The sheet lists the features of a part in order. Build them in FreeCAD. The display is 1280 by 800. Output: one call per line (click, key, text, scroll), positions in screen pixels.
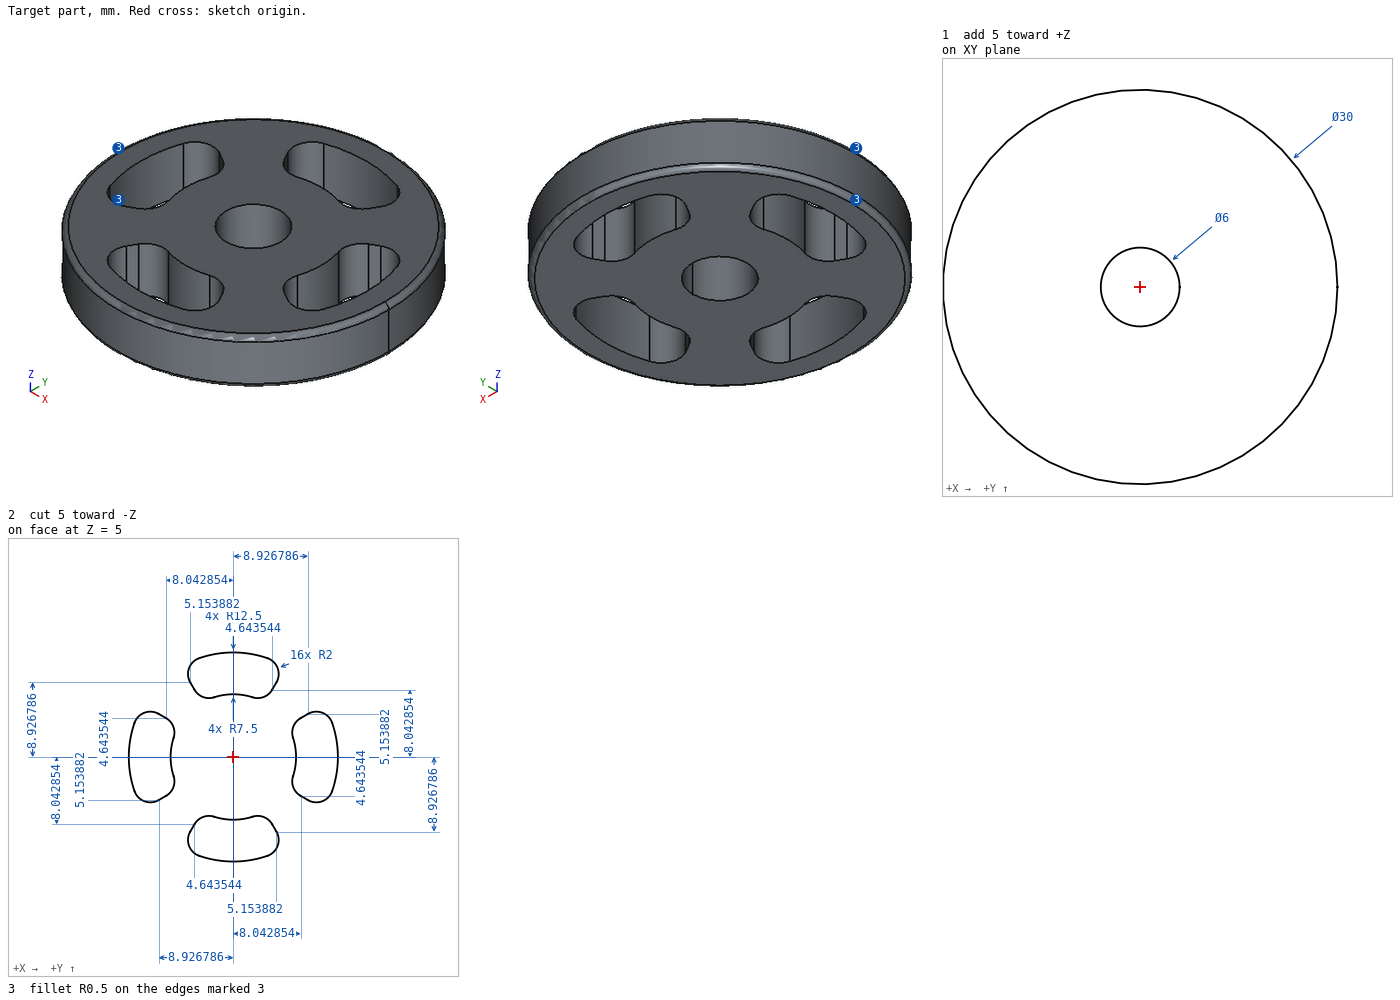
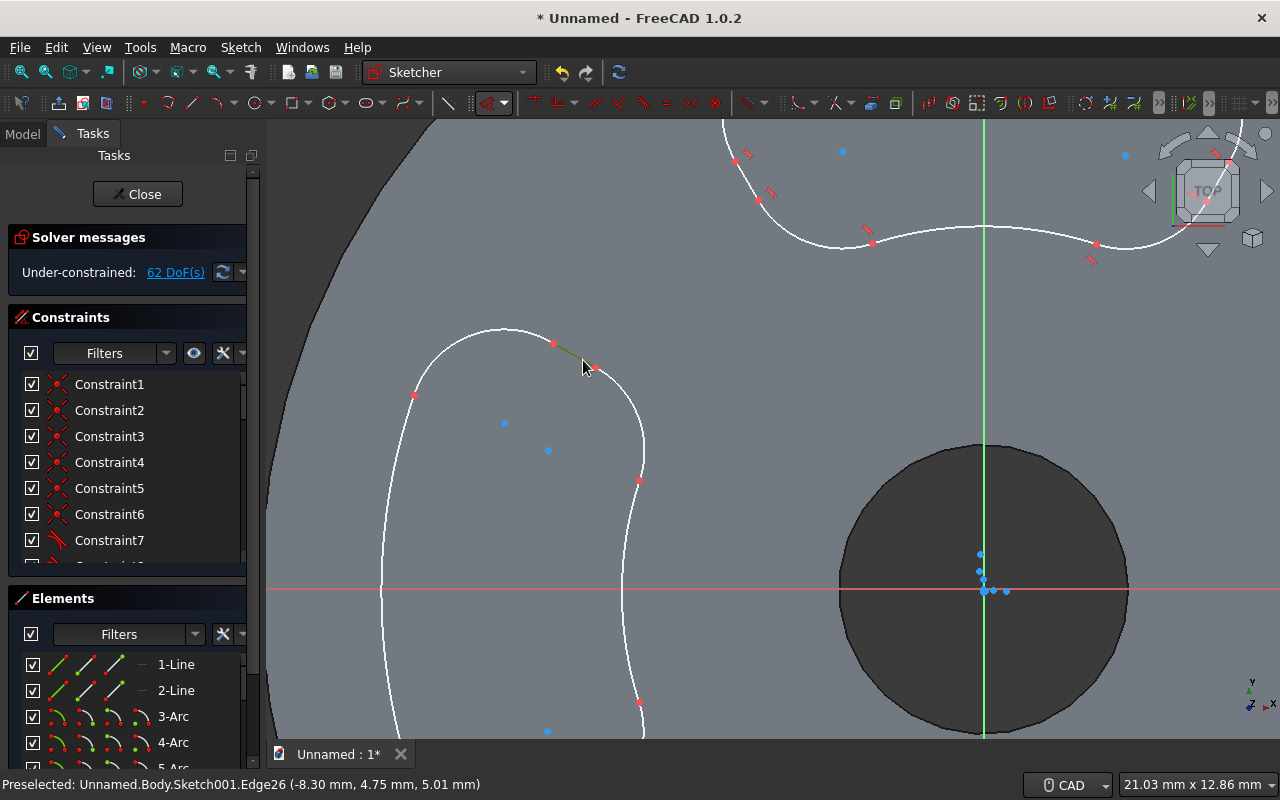
click(644, 441)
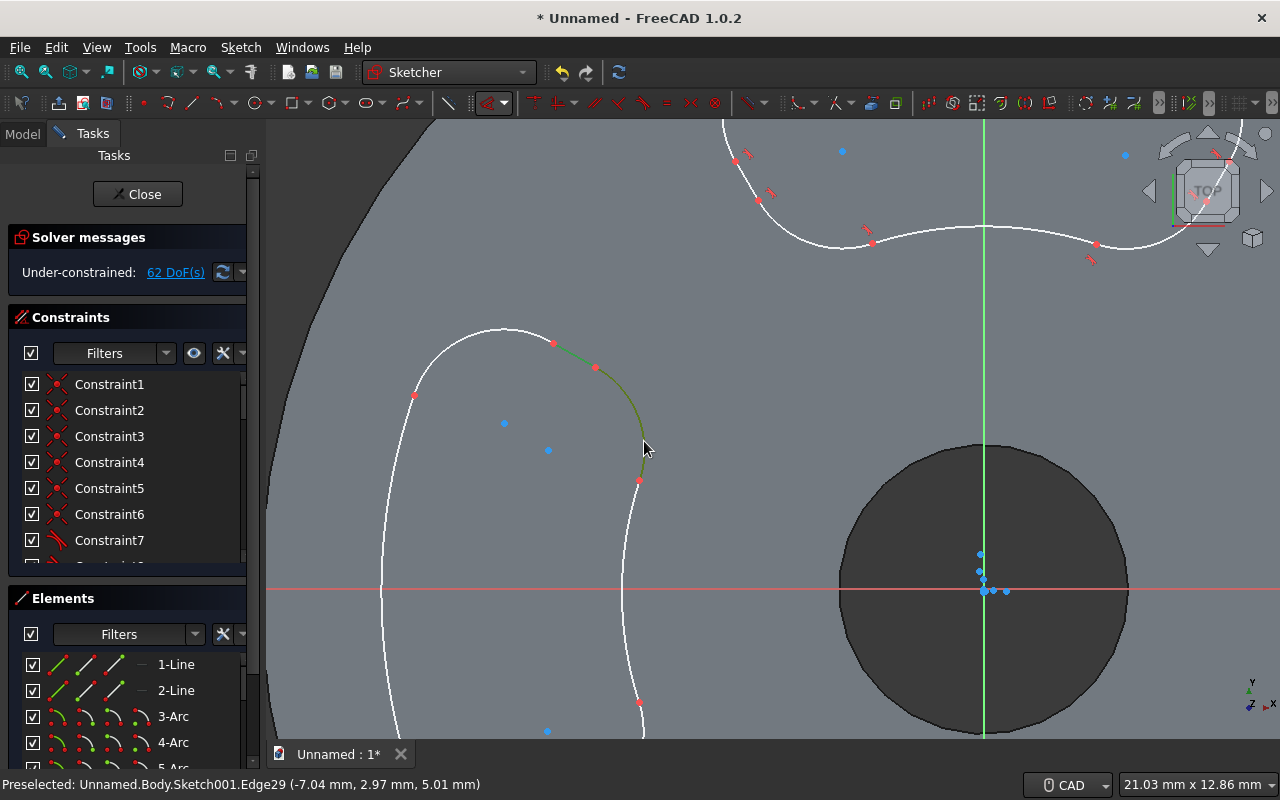
click(644, 104)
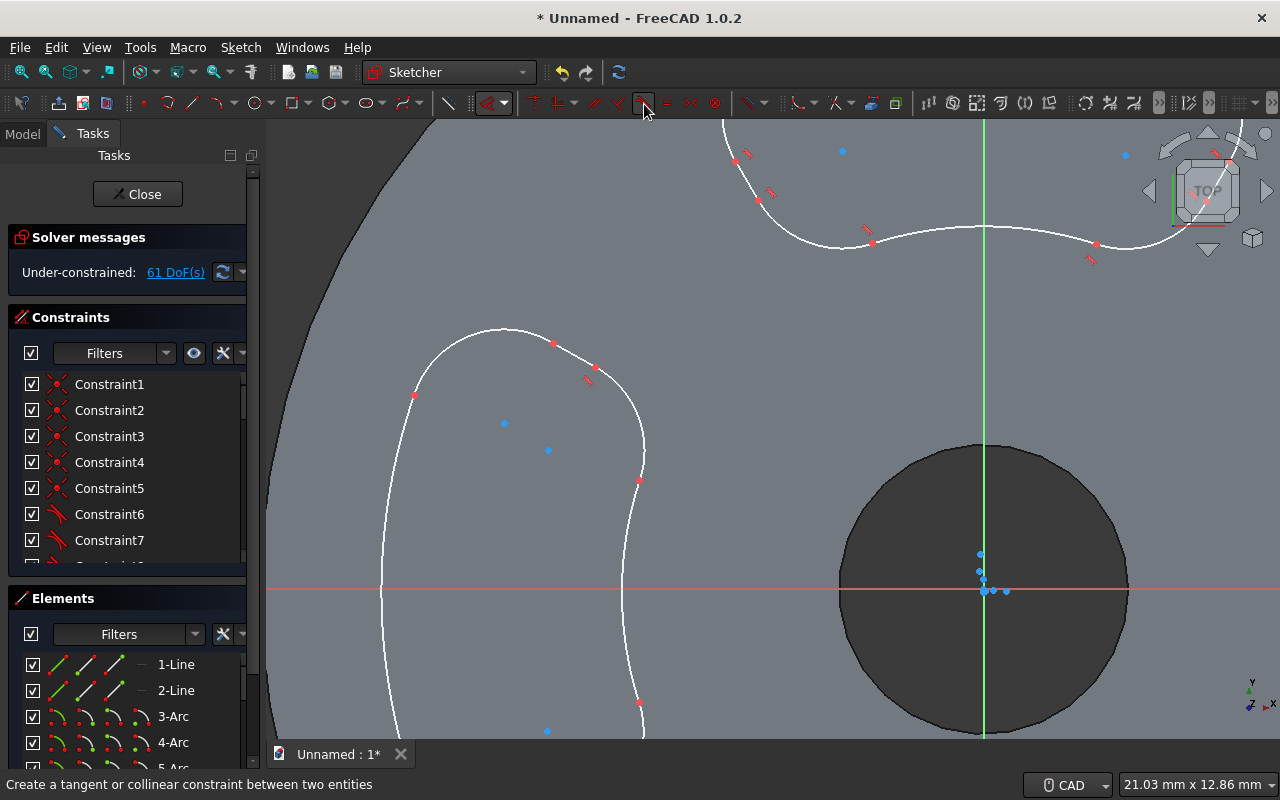
click(583, 360)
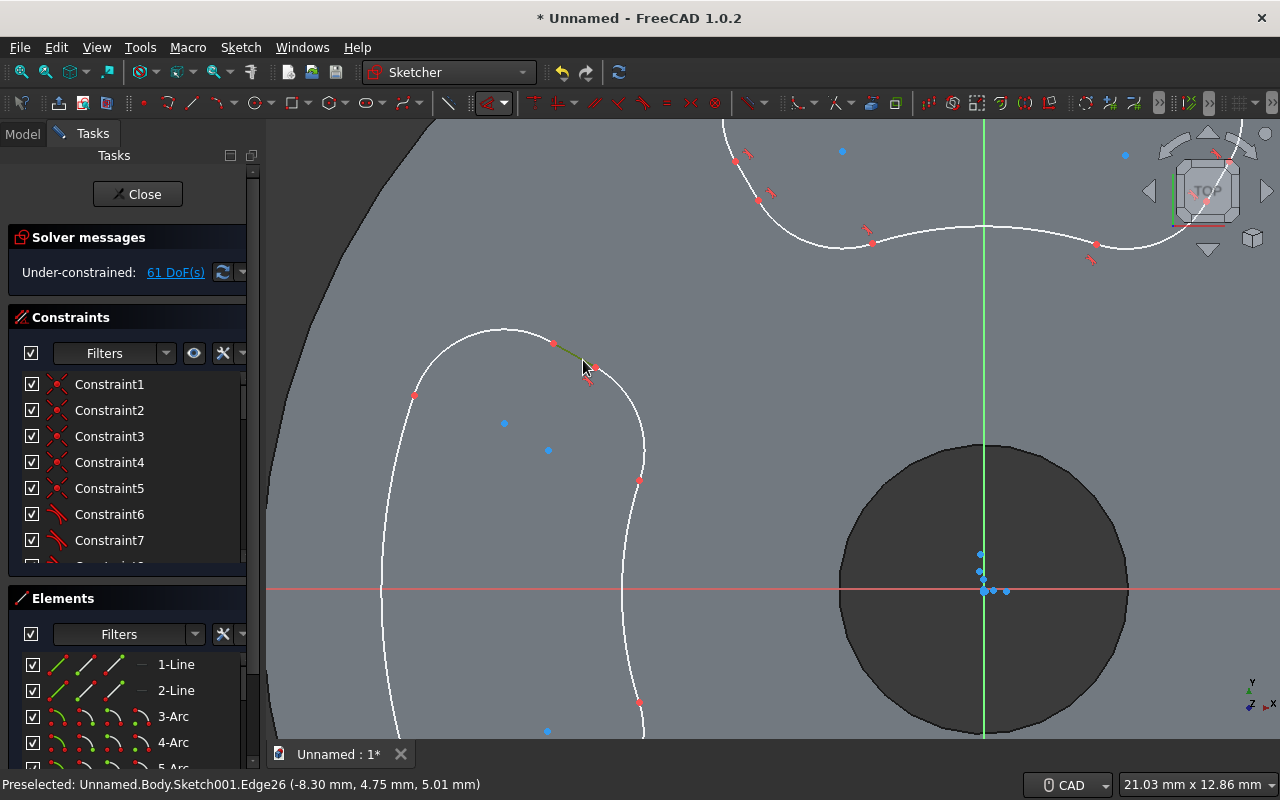
click(505, 329)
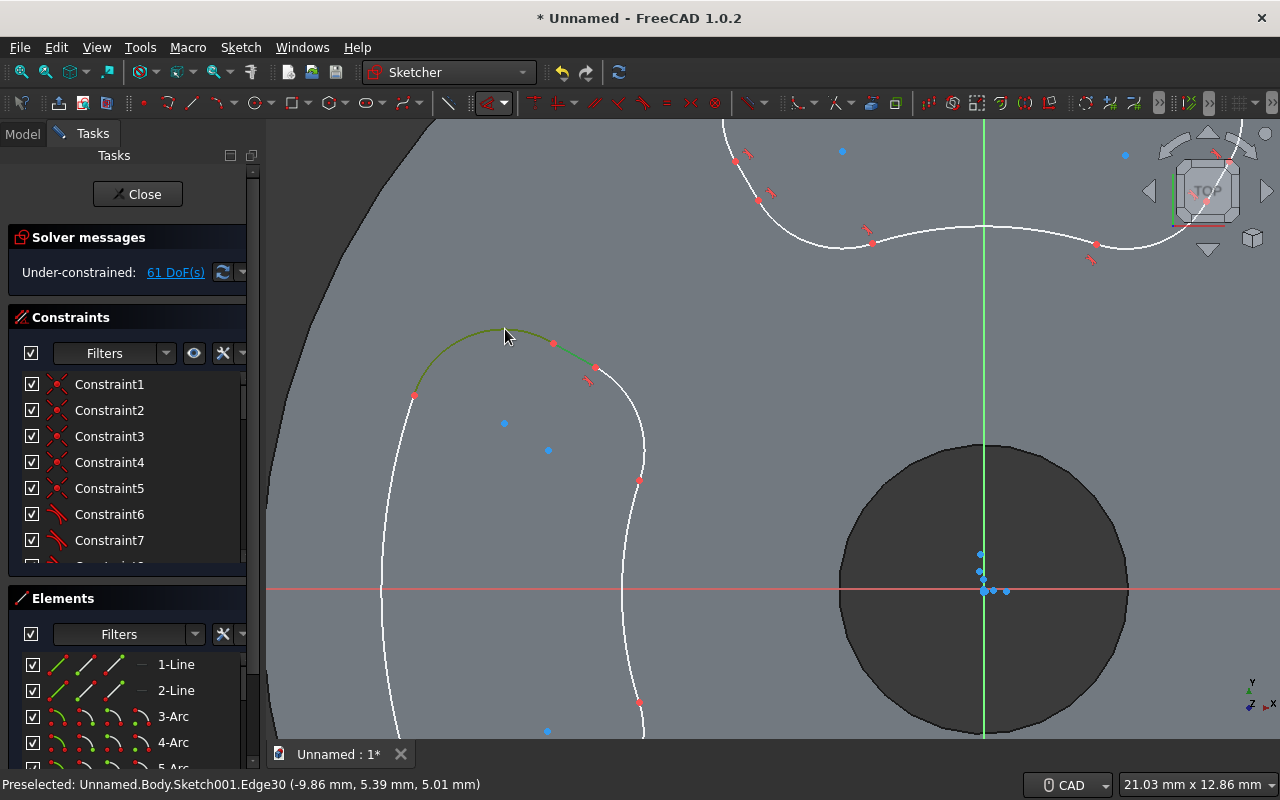
click(644, 104)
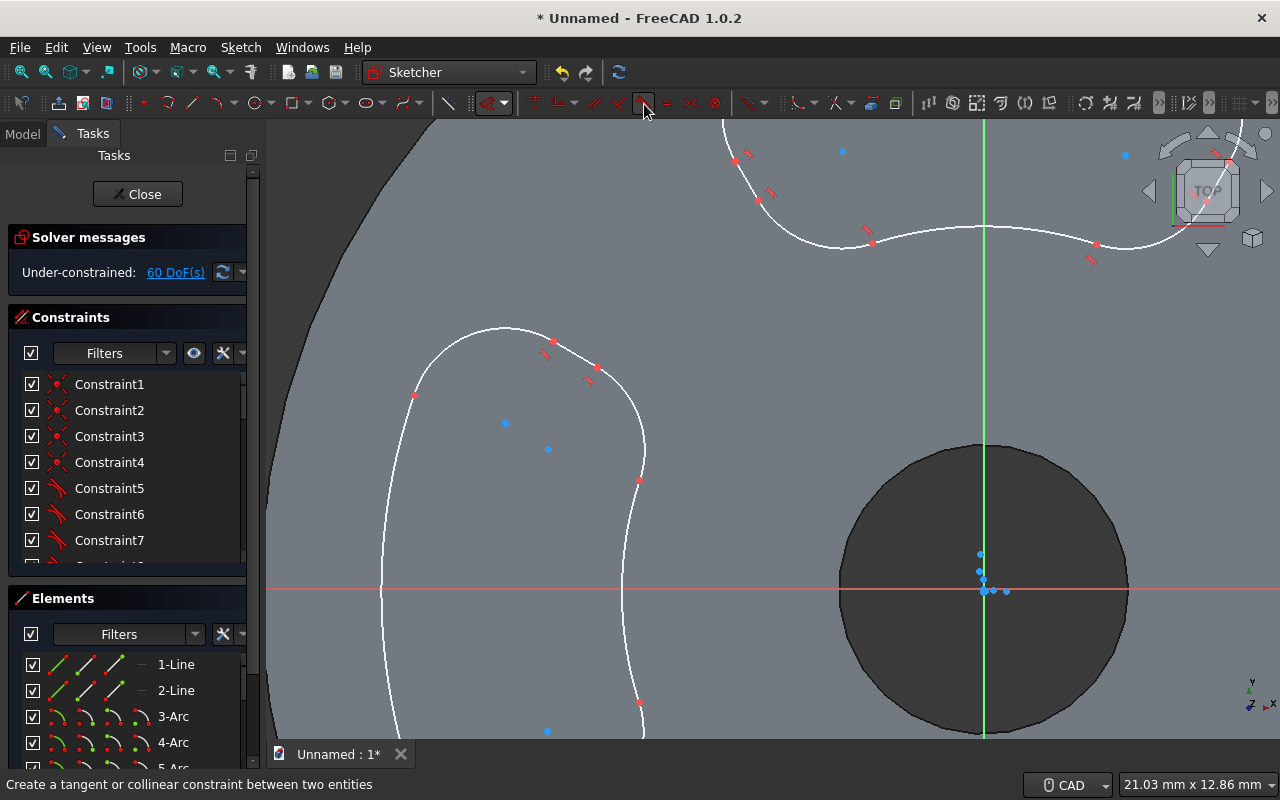
scroll(584, 360, down, 6)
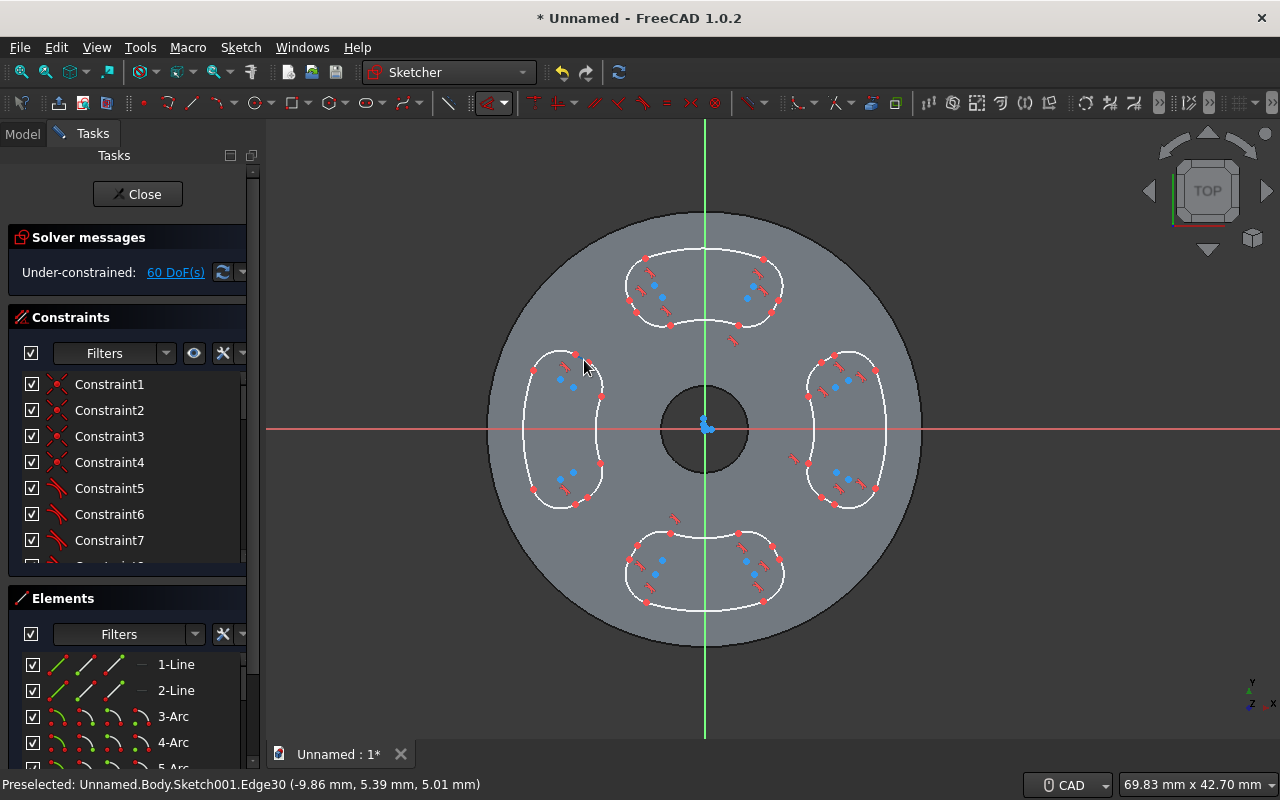
click(596, 490)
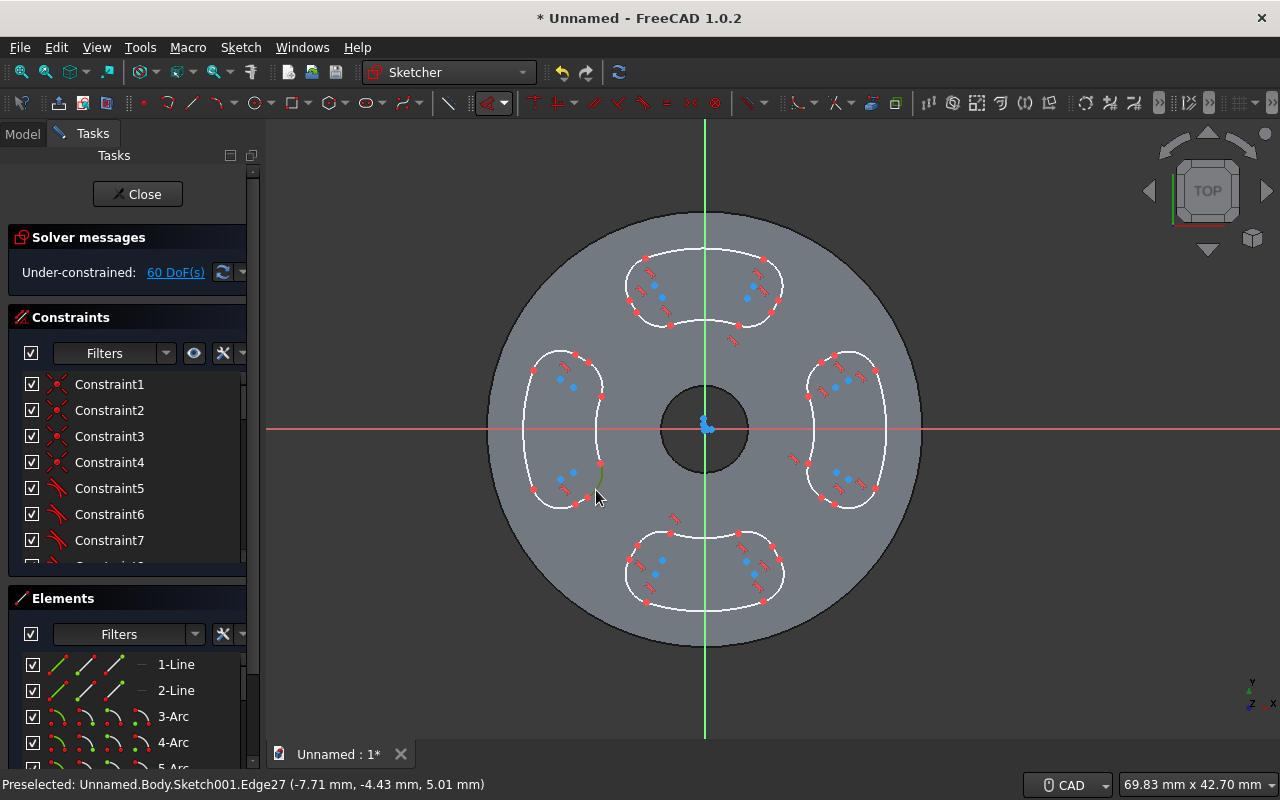
click(597, 416)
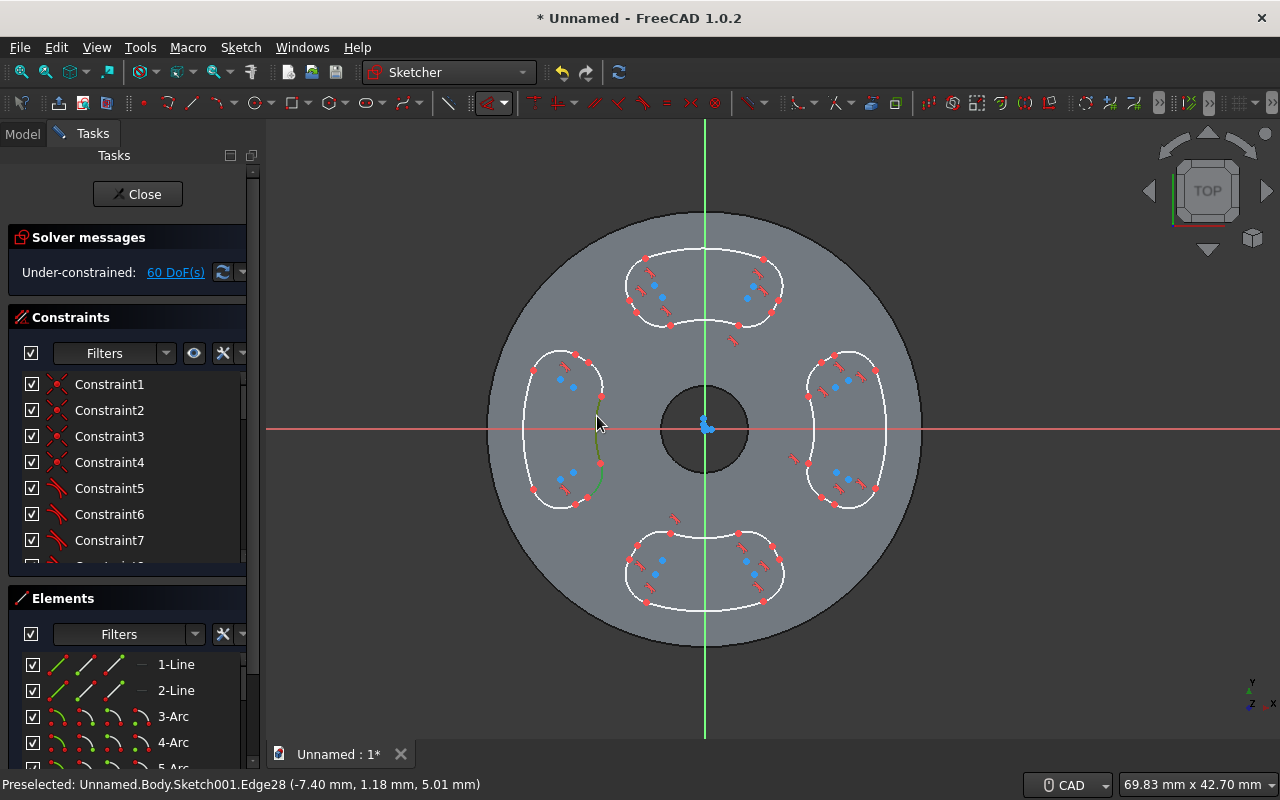
click(644, 104)